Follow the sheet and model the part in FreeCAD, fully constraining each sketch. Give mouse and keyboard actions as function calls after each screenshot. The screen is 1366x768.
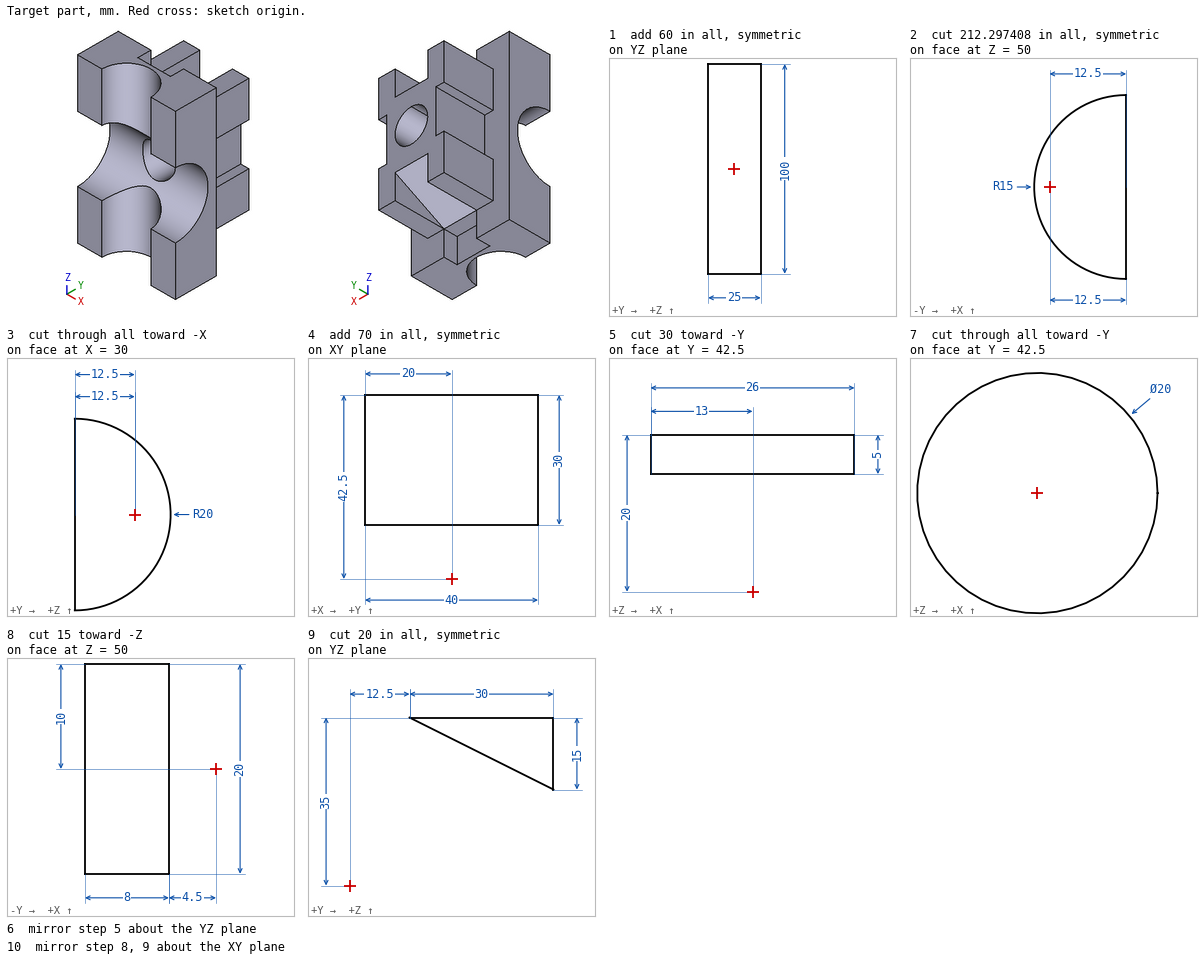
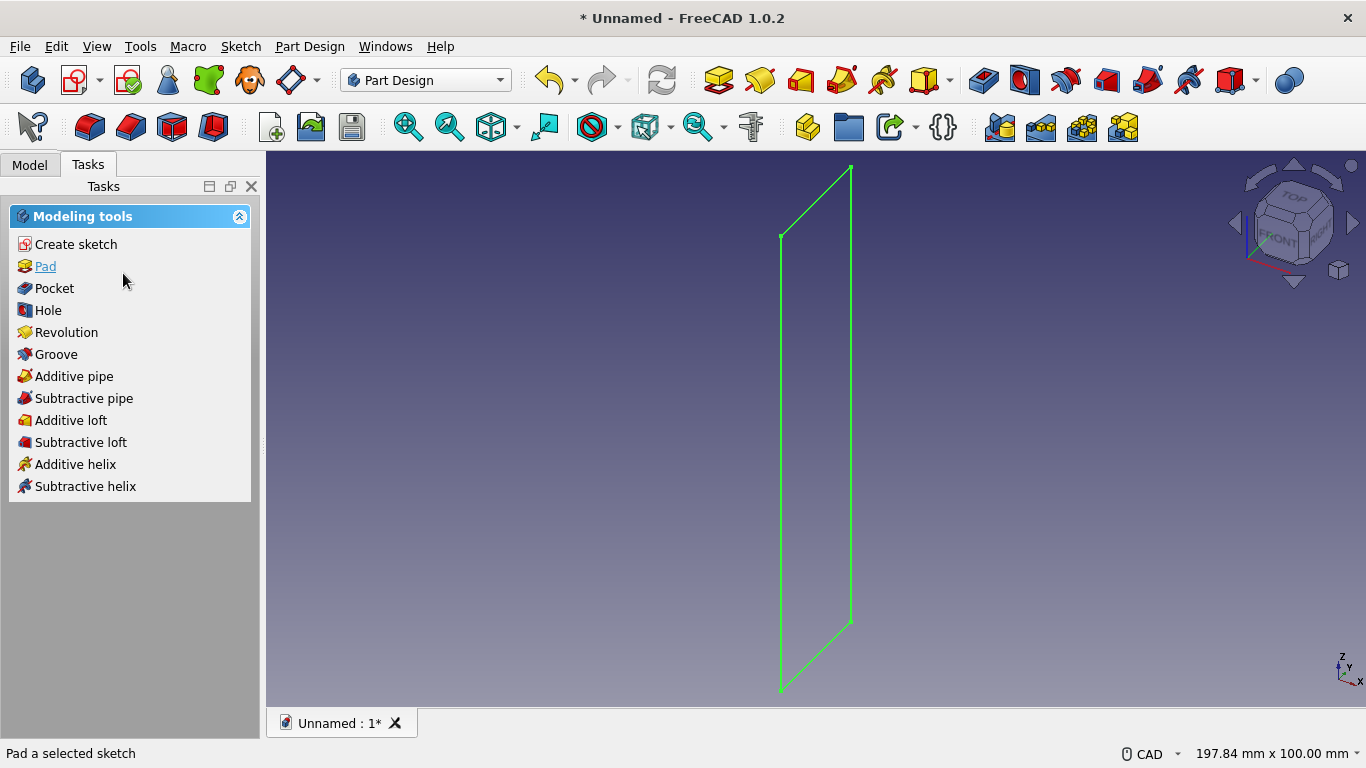
click(719, 80)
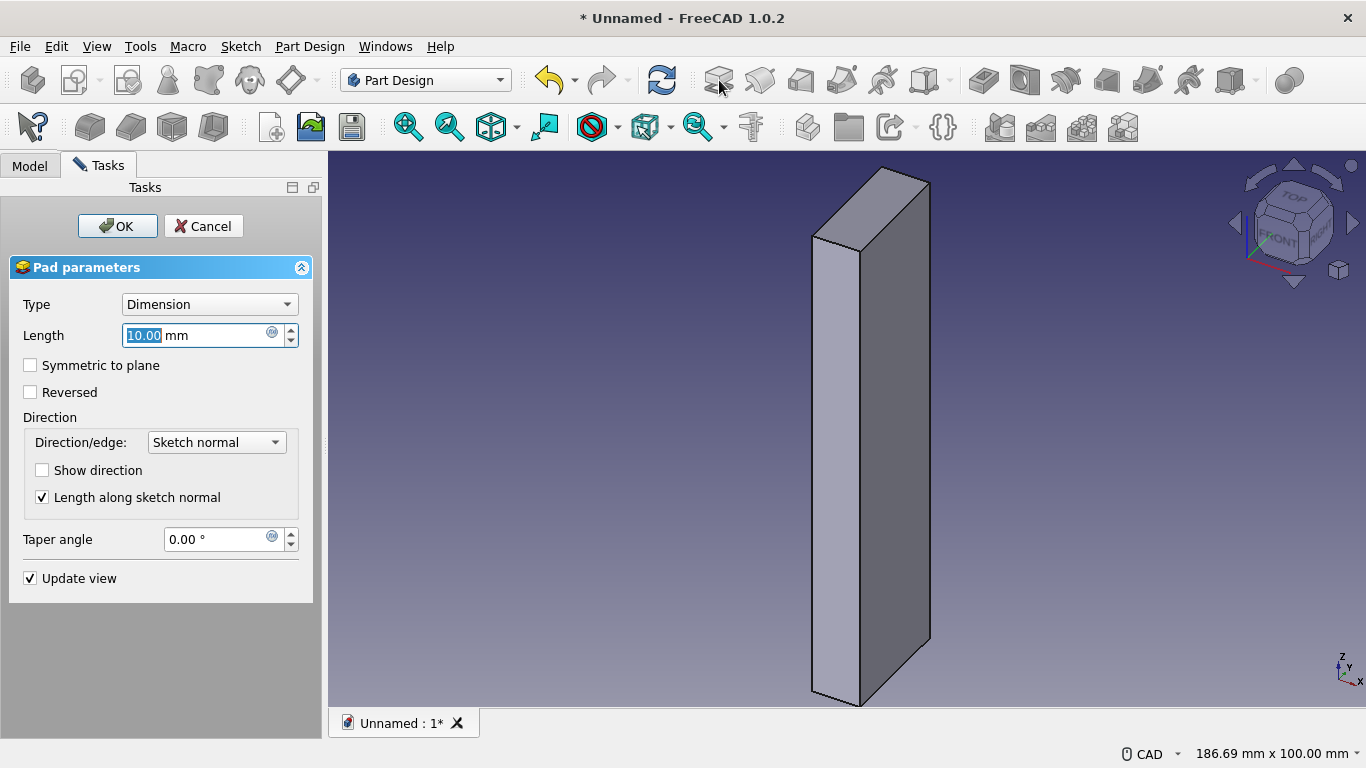
text(60)
key(Tab)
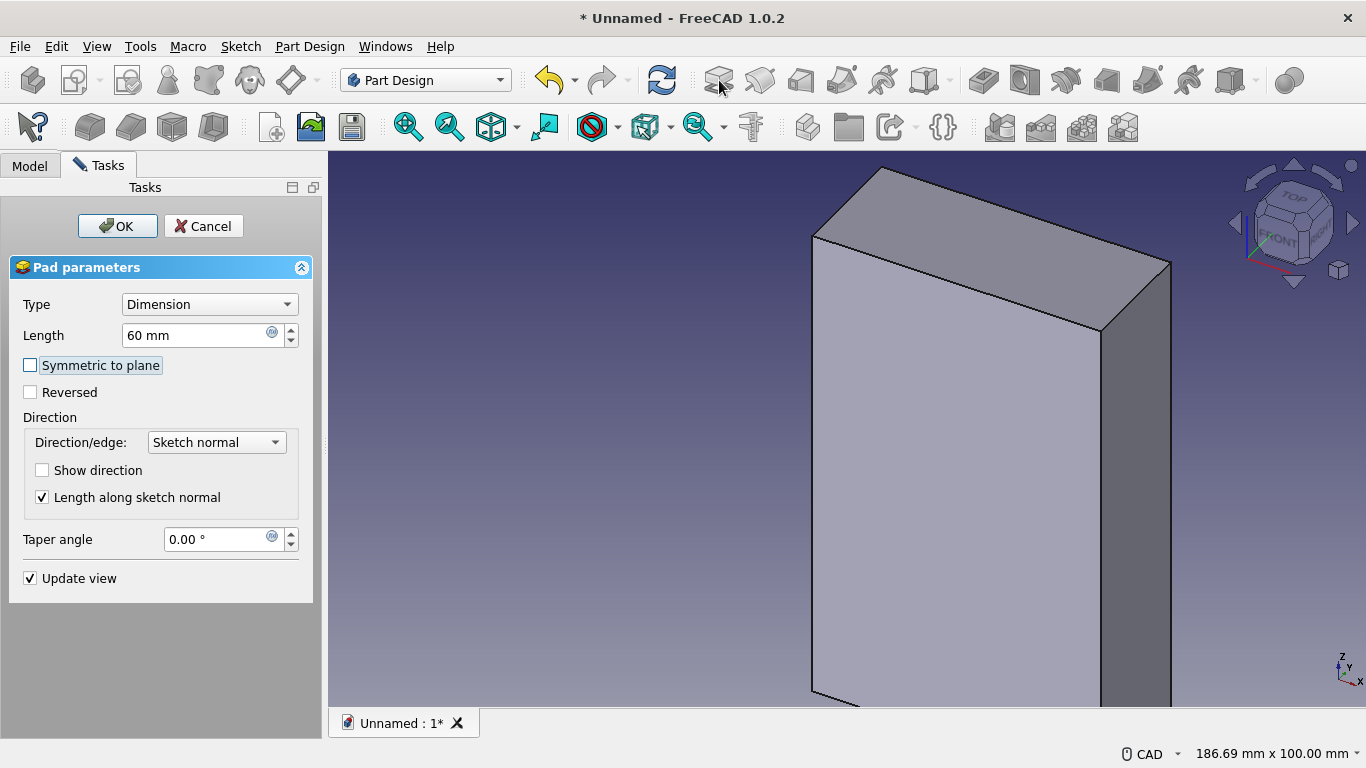
click(31, 365)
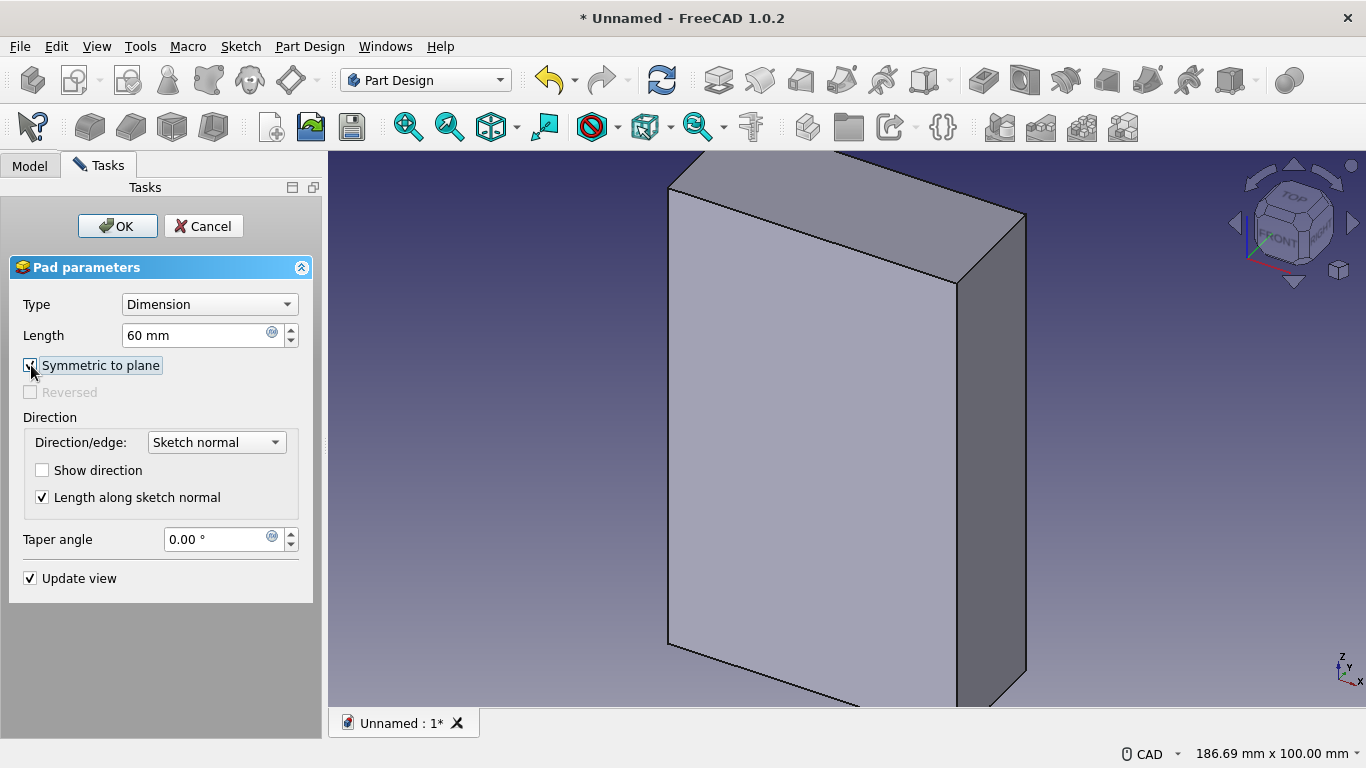
click(118, 226)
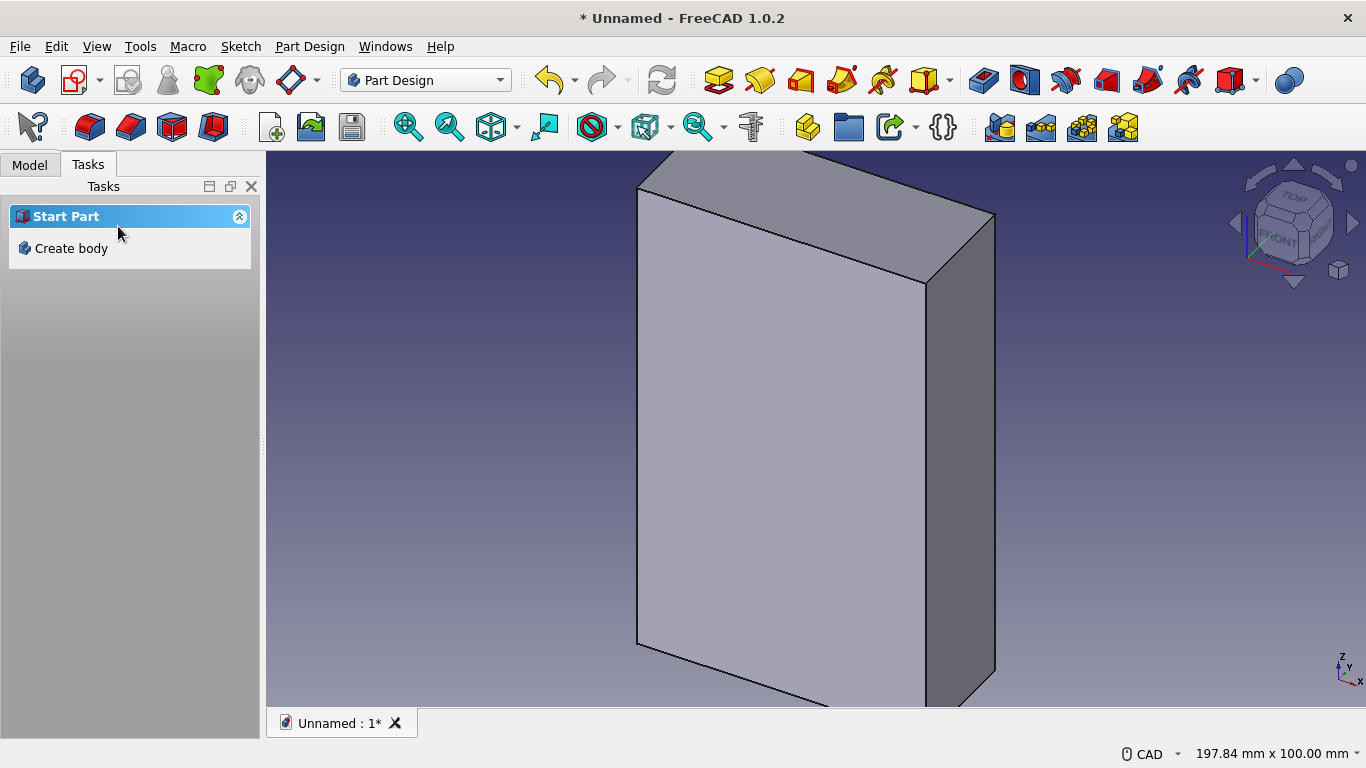
click(409, 128)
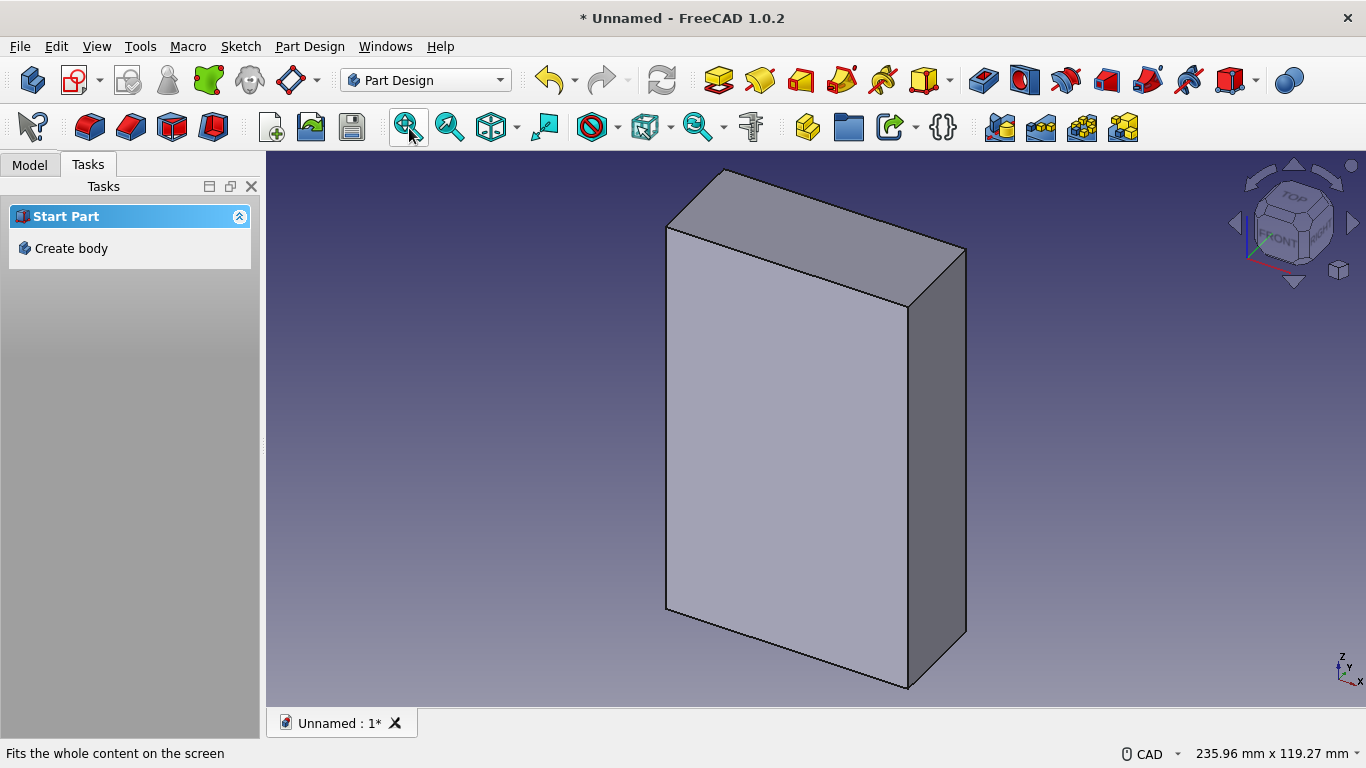
click(816, 237)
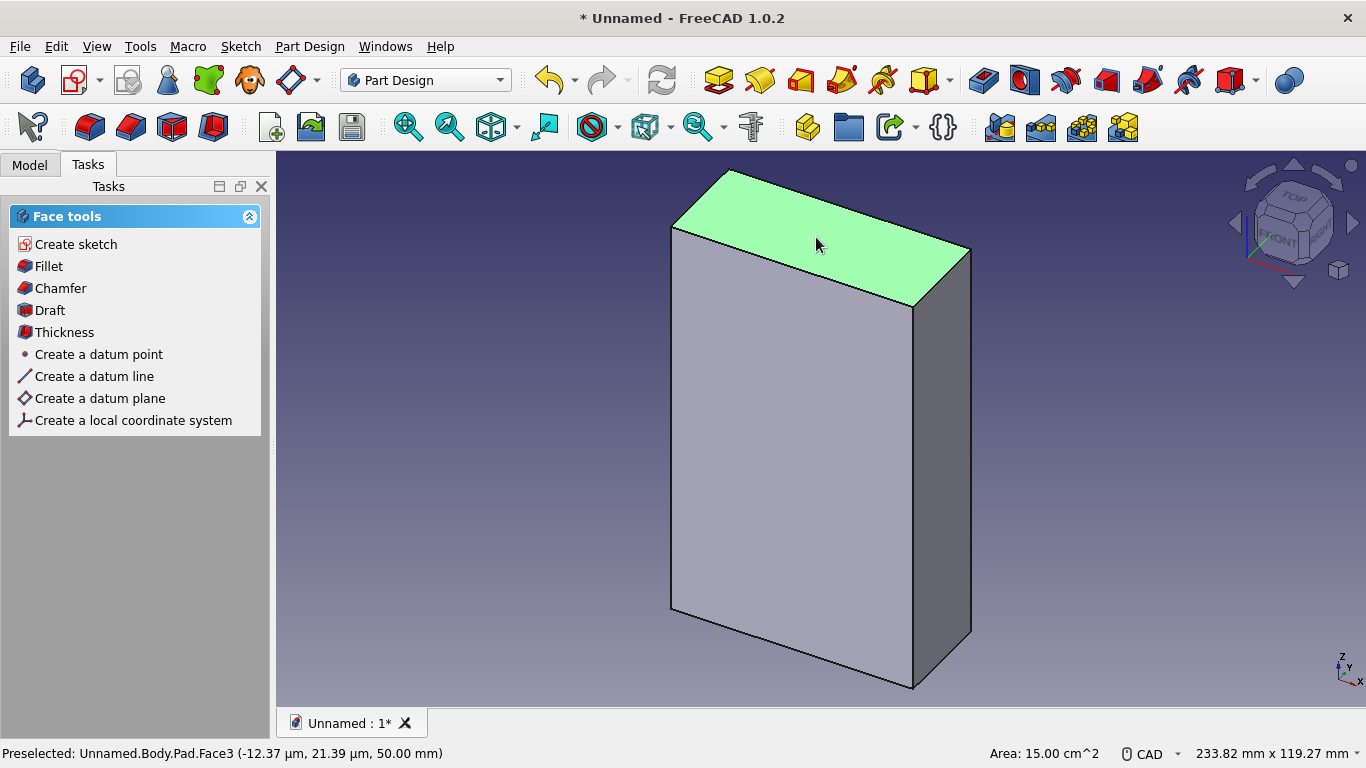
click(74, 80)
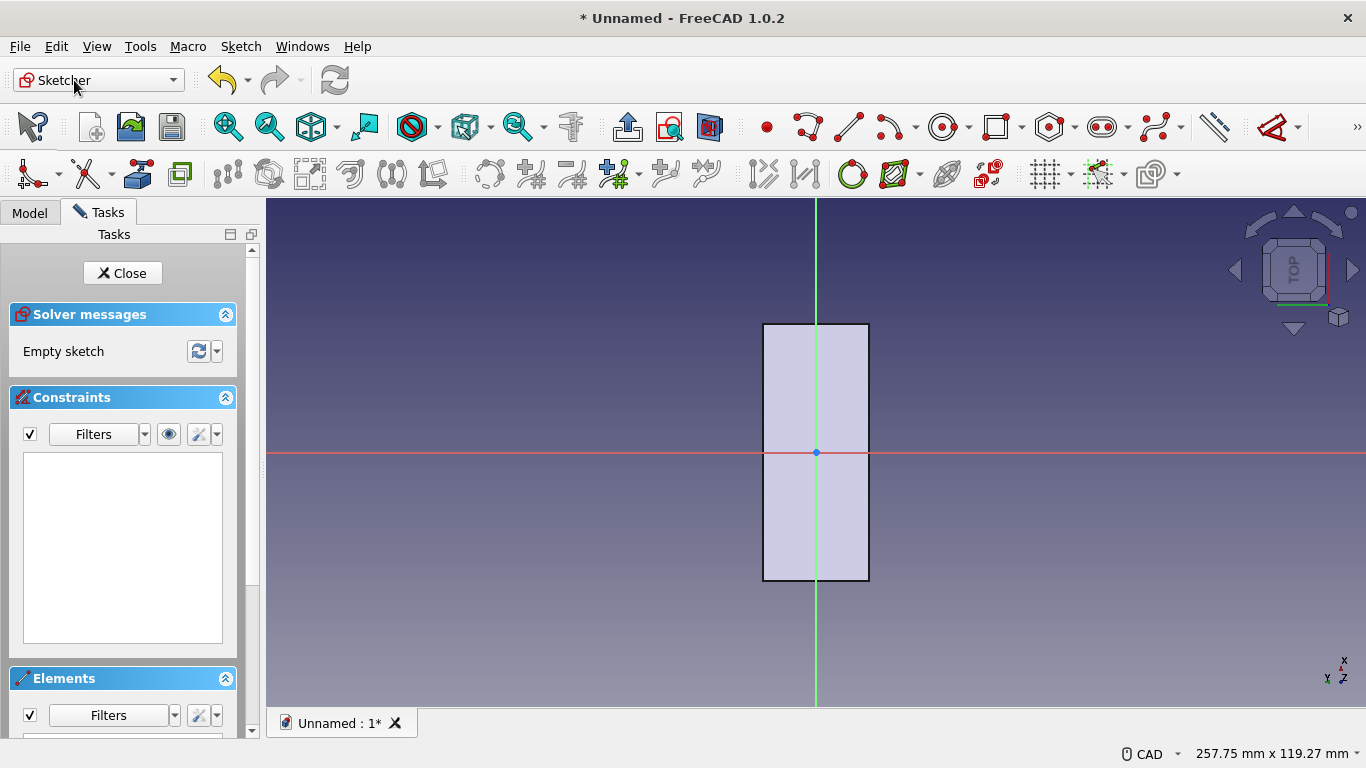
scroll(890, 453, up, 5)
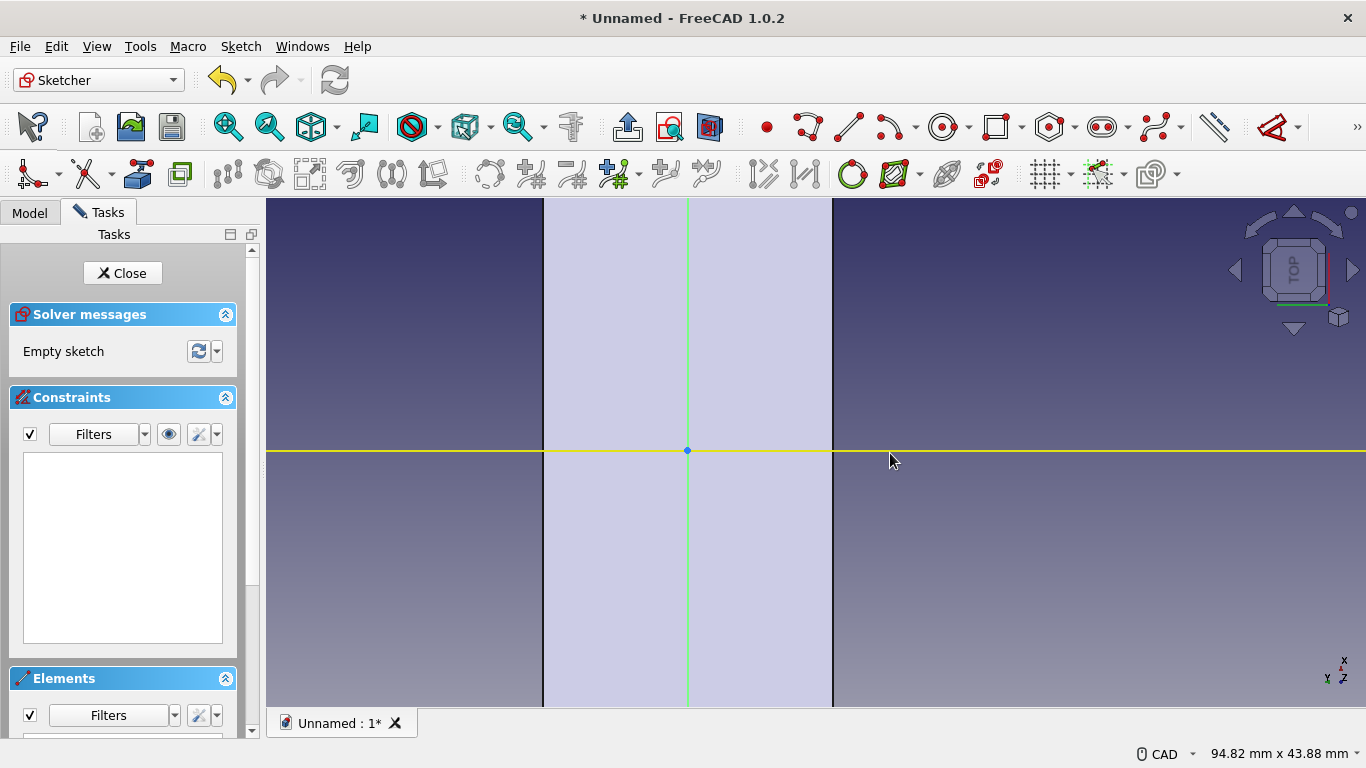
key(g)
key(l)